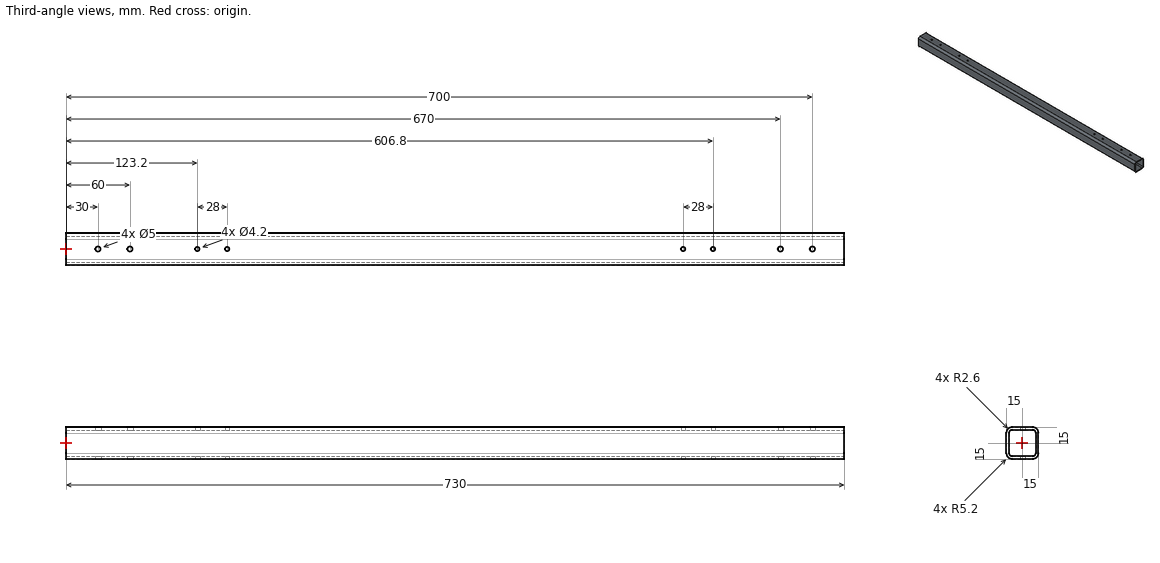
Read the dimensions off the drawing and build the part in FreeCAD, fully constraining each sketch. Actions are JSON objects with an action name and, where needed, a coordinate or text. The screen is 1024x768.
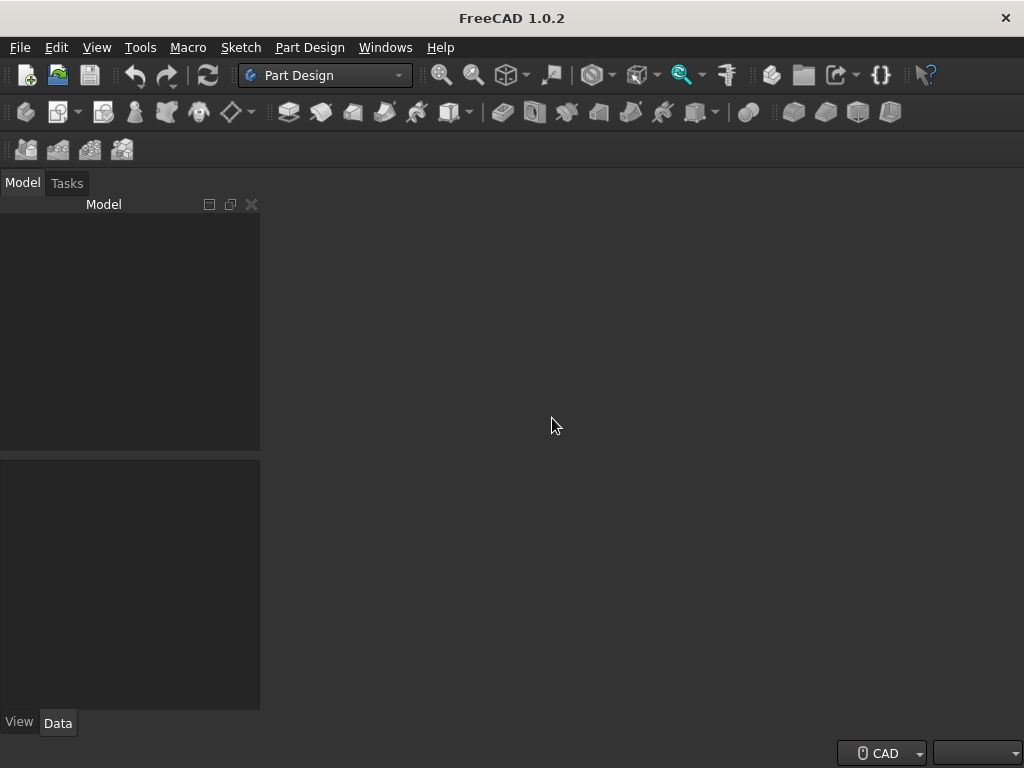
{"action": "left_click", "coordinate": [26, 76]}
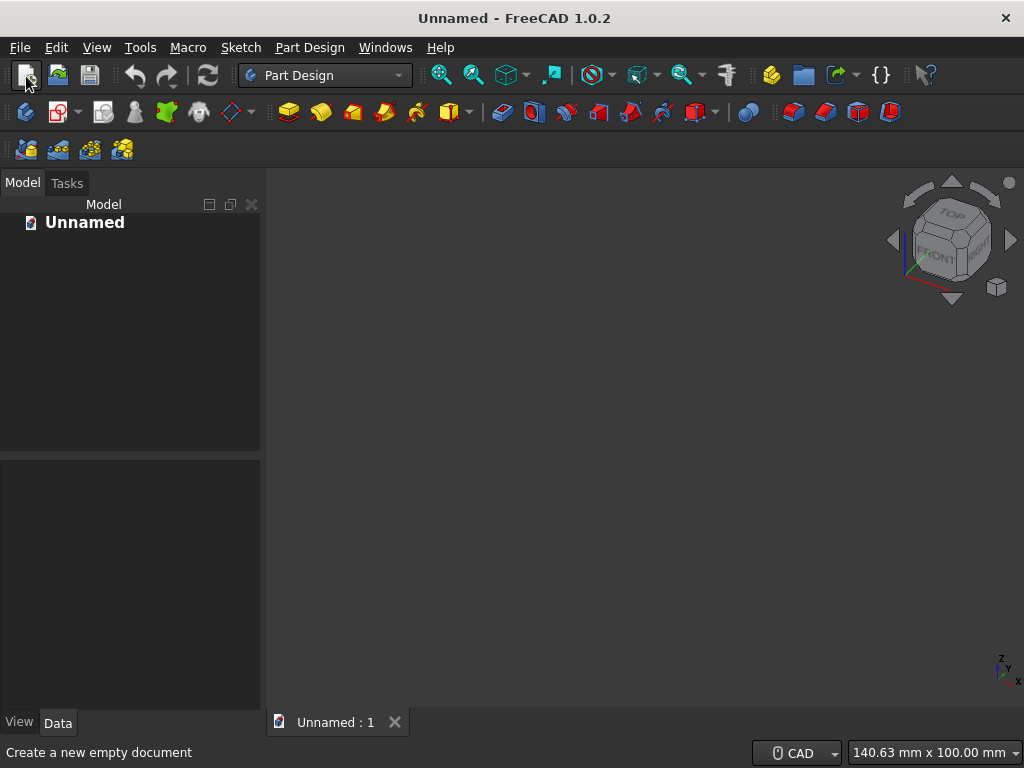
{"action": "left_click", "coordinate": [58, 112]}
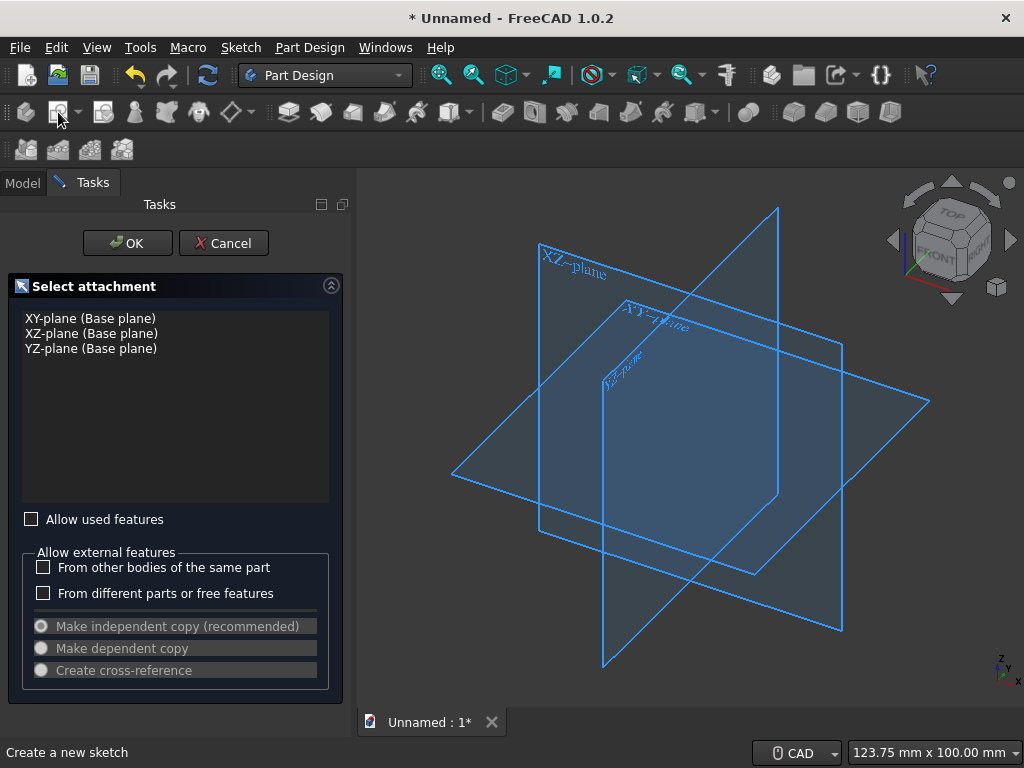
{"action": "left_click", "coordinate": [82, 348]}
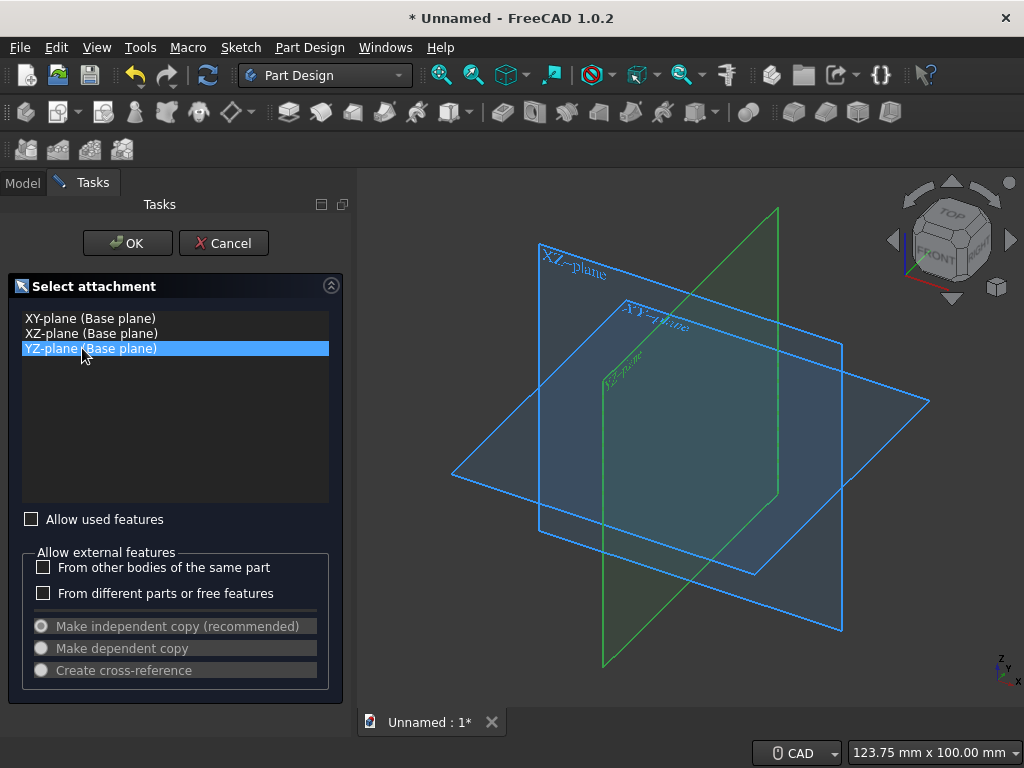
{"action": "left_click", "coordinate": [128, 243]}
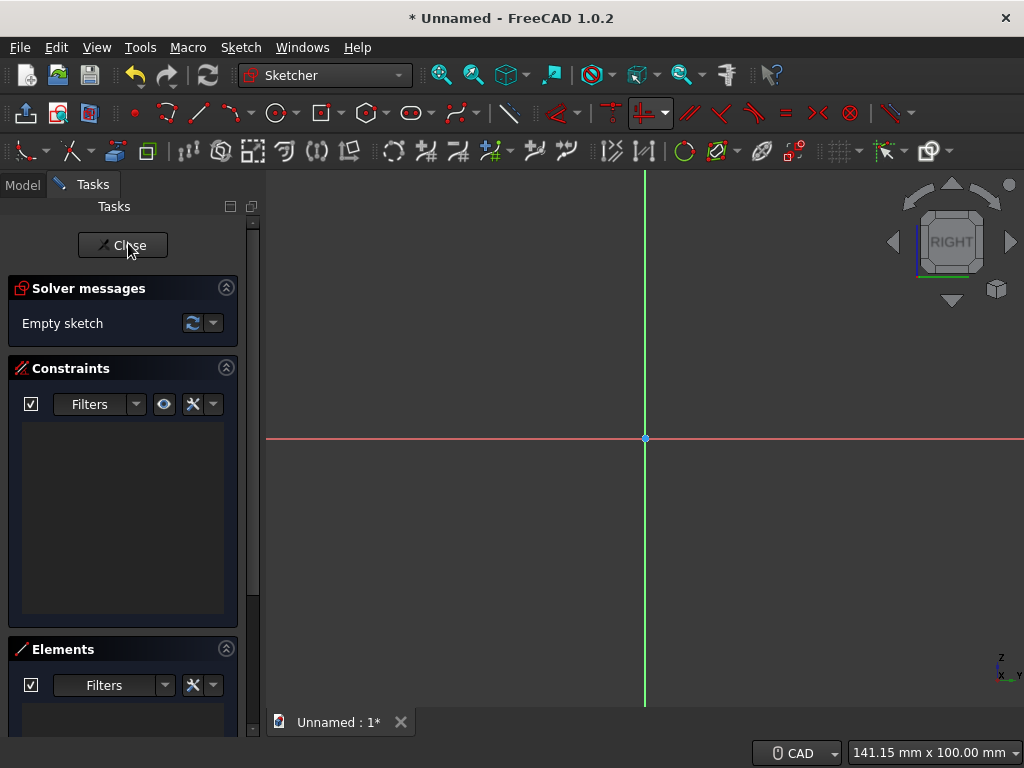
{"action": "scroll", "coordinate": [701, 438], "scroll_direction": "up", "scroll_amount": 4}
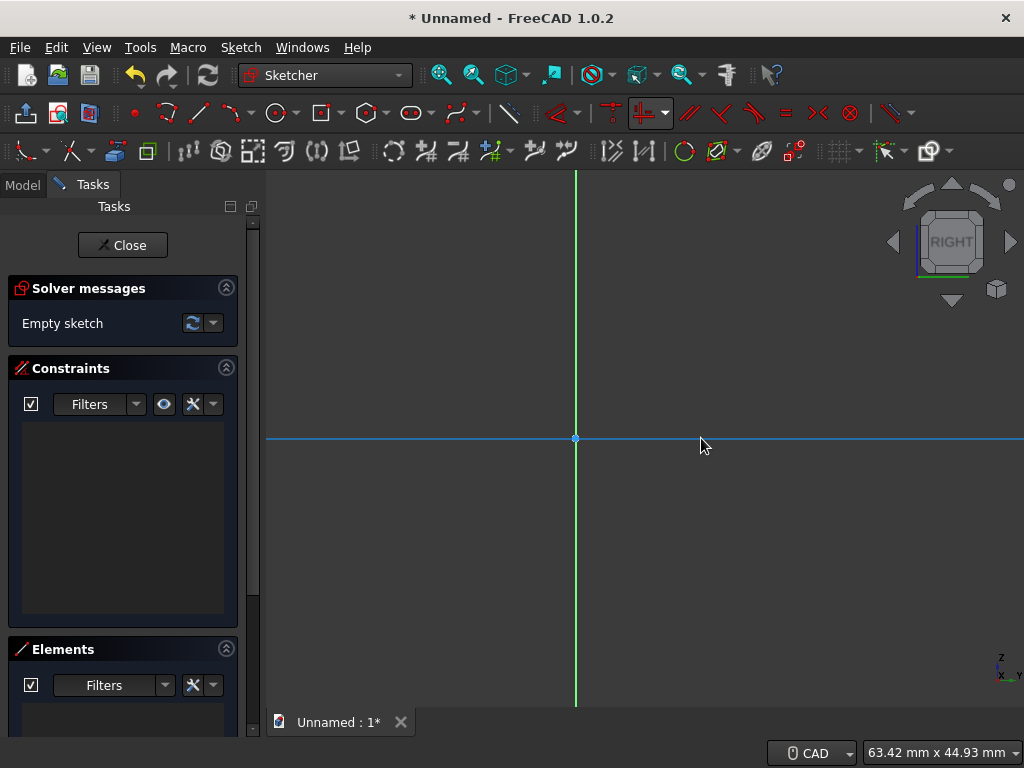
{"action": "left_click", "coordinate": [200, 114]}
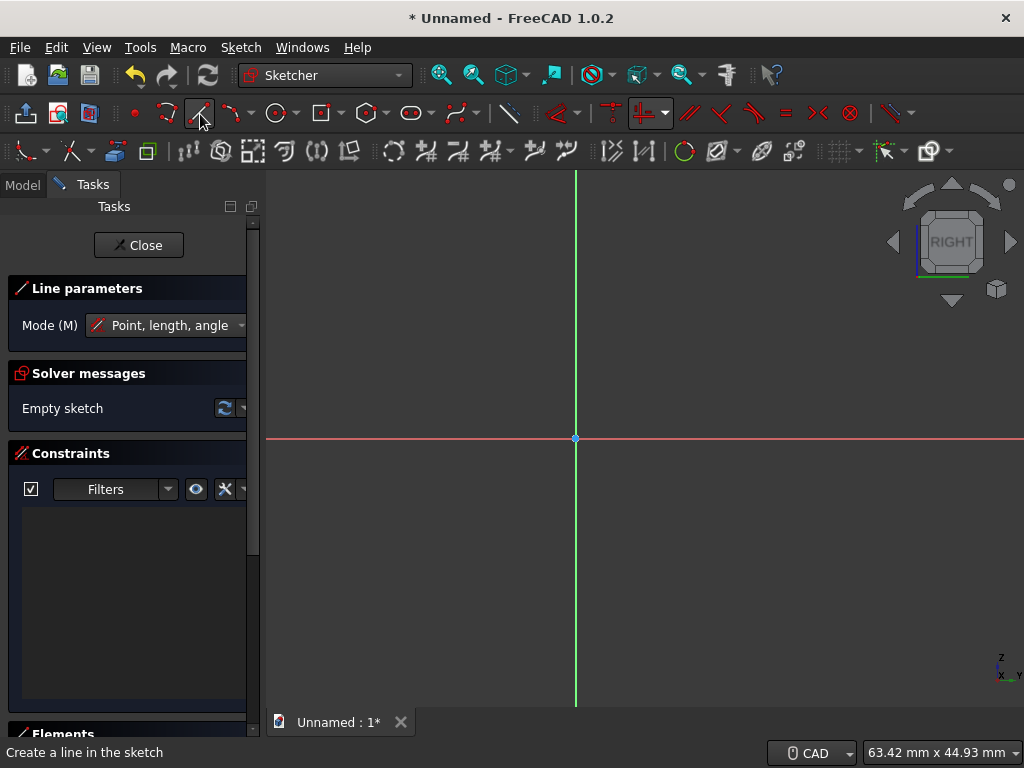
{"action": "left_click", "coordinate": [396, 321]}
{"action": "left_click", "coordinate": [396, 556]}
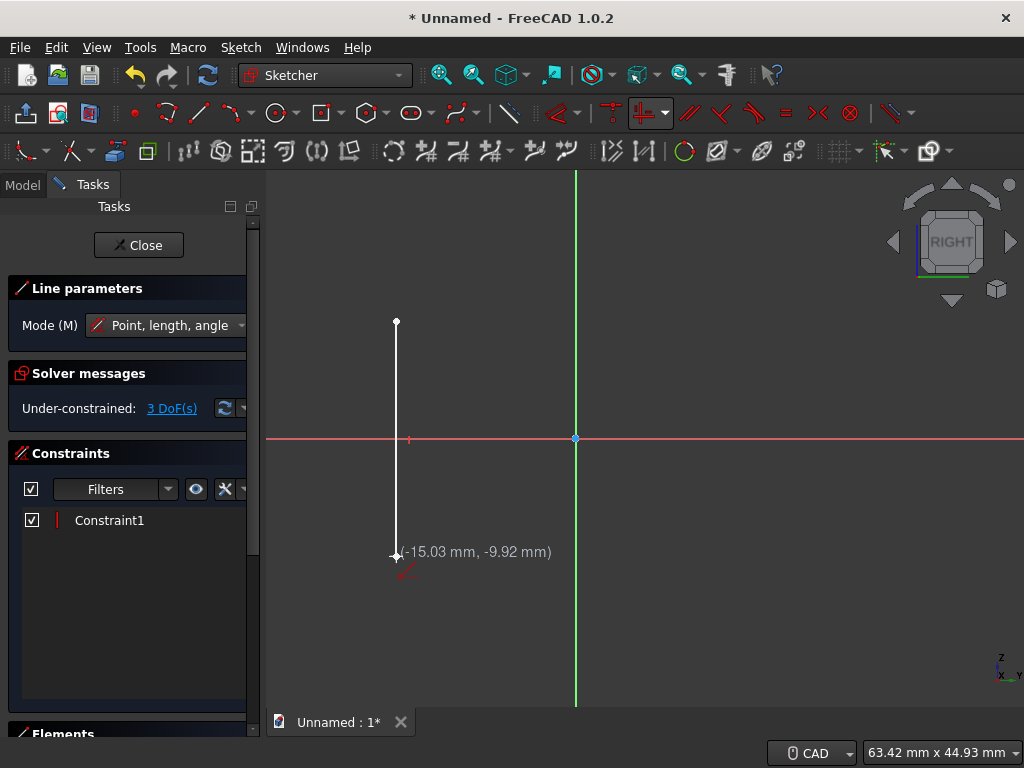
{"action": "left_click", "coordinate": [459, 618]}
{"action": "left_click", "coordinate": [693, 618]}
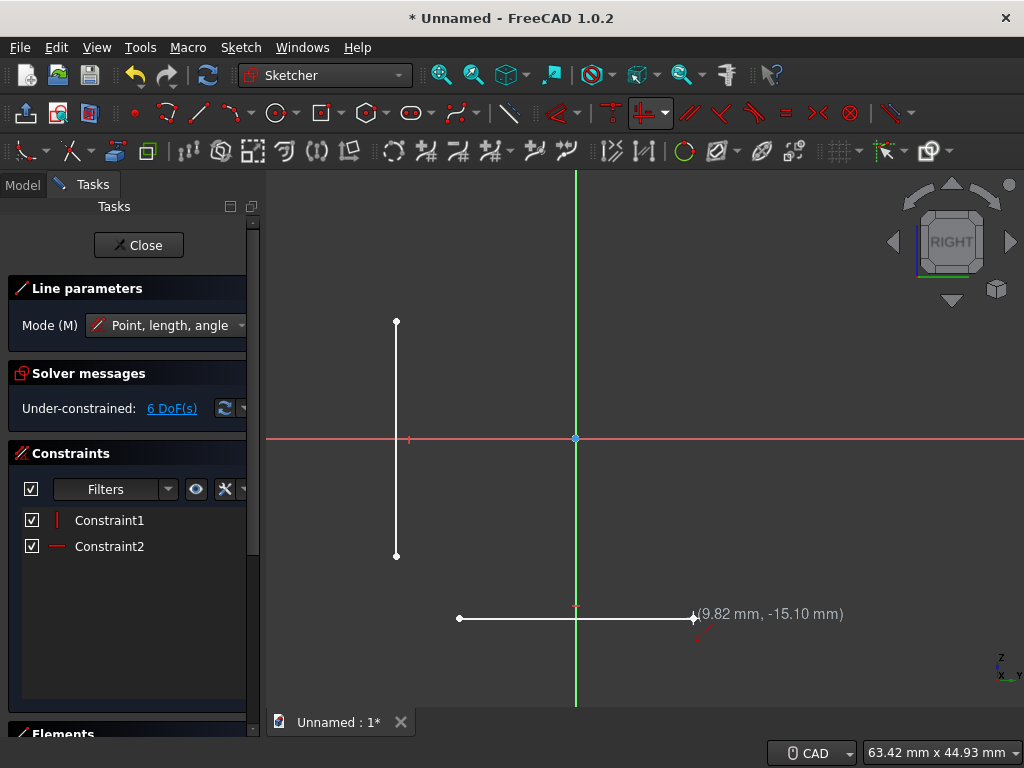
{"action": "left_click", "coordinate": [755, 556]}
{"action": "left_click", "coordinate": [755, 321]}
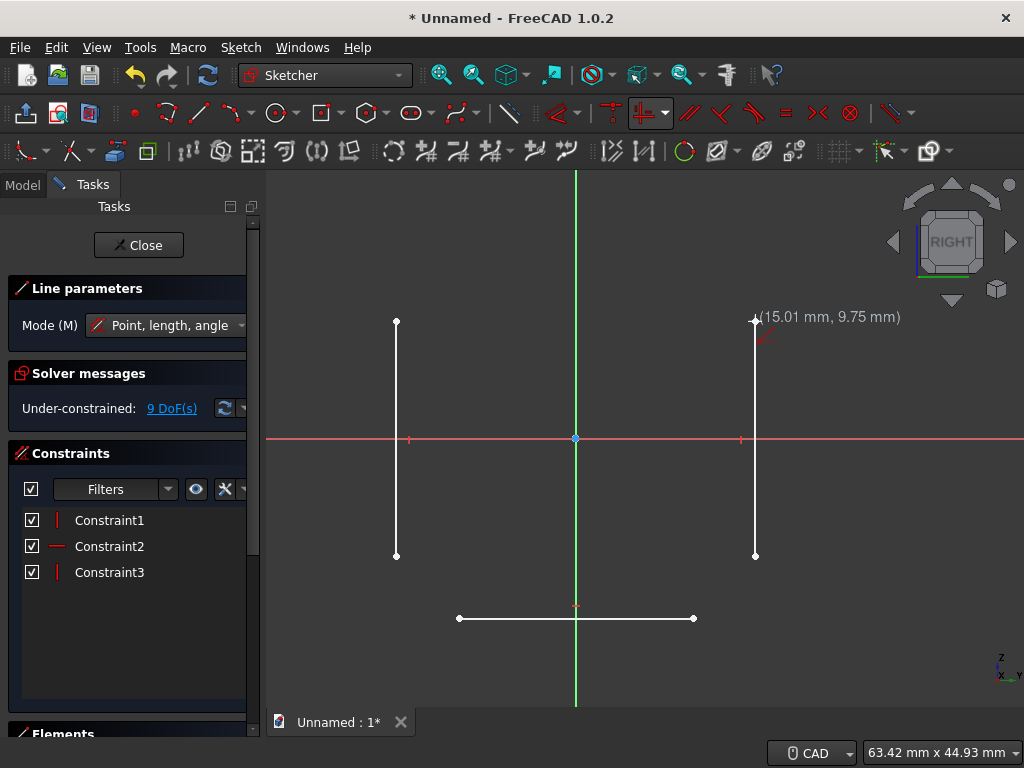
{"action": "left_click", "coordinate": [693, 259]}
{"action": "left_click", "coordinate": [459, 259]}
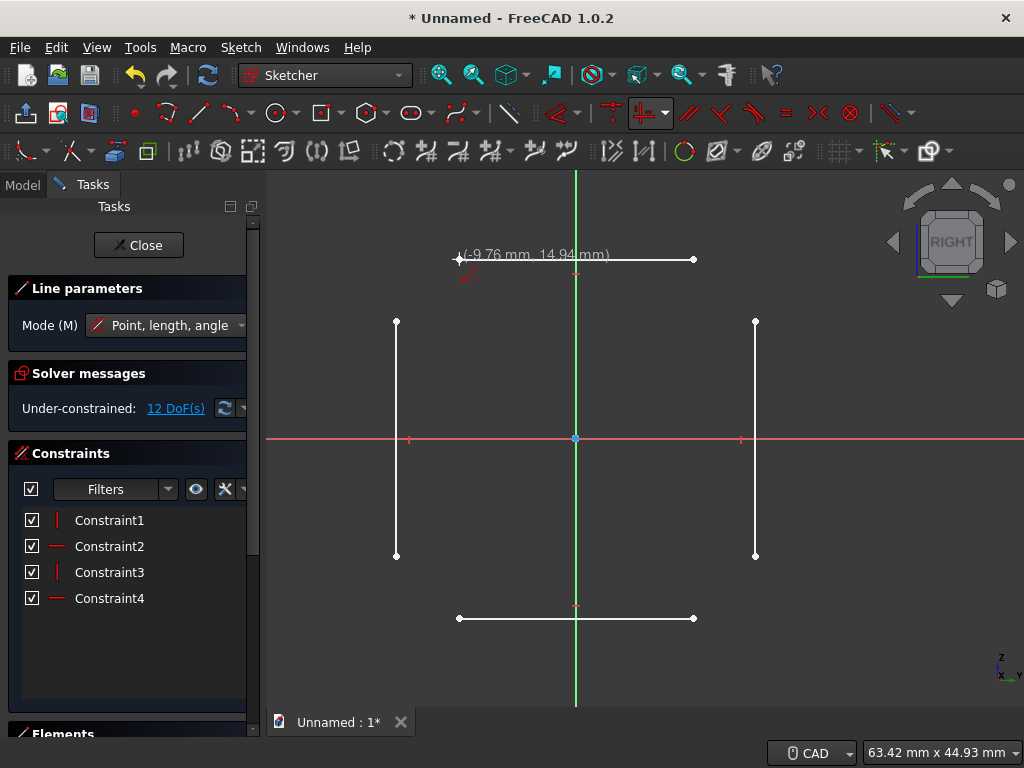
{"action": "left_click", "coordinate": [232, 114]}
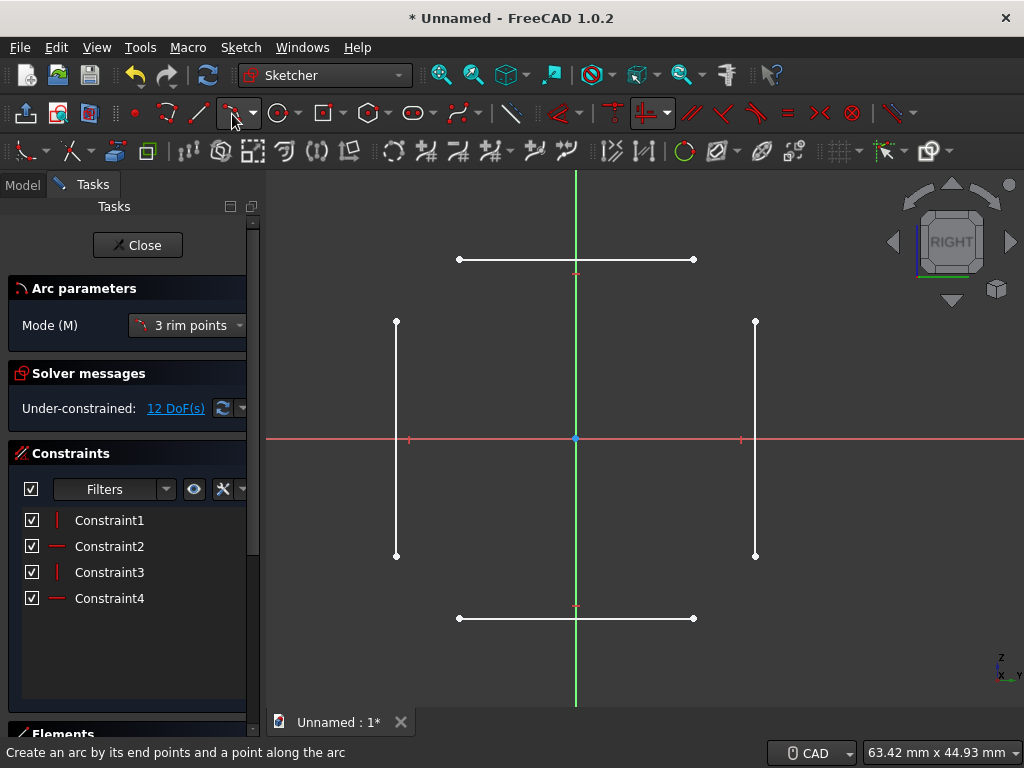
{"action": "left_click", "coordinate": [396, 557]}
{"action": "left_click", "coordinate": [459, 619]}
{"action": "left_click", "coordinate": [415, 600]}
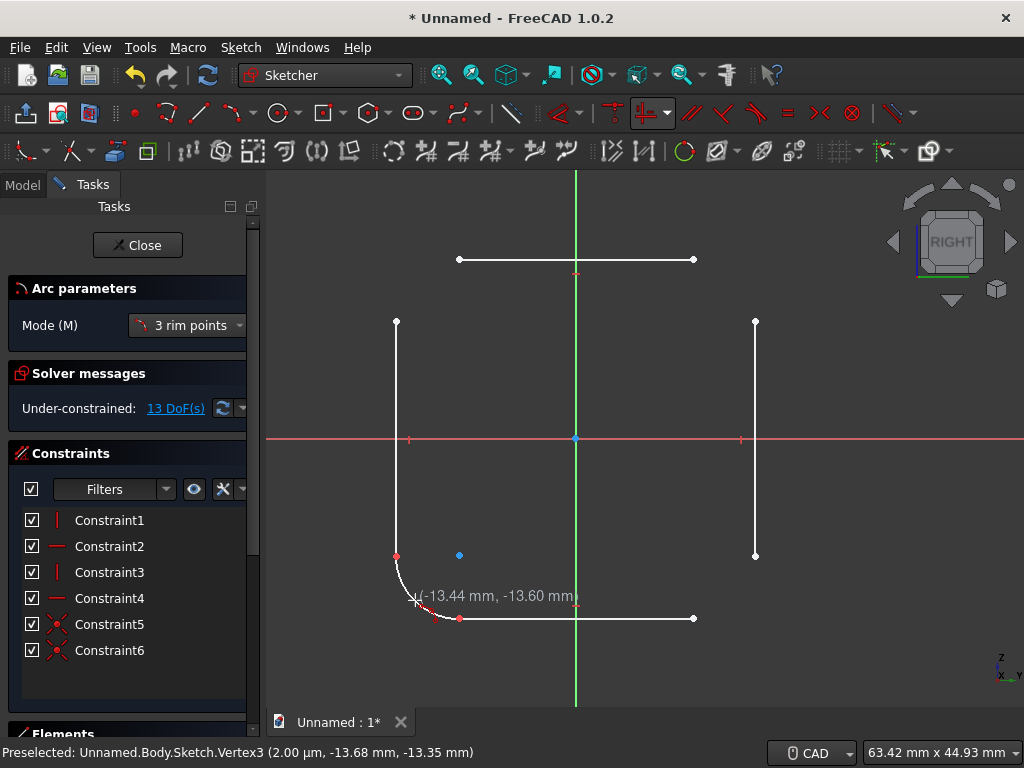
{"action": "left_click", "coordinate": [693, 619]}
{"action": "left_click", "coordinate": [755, 557]}
{"action": "left_click", "coordinate": [737, 600]}